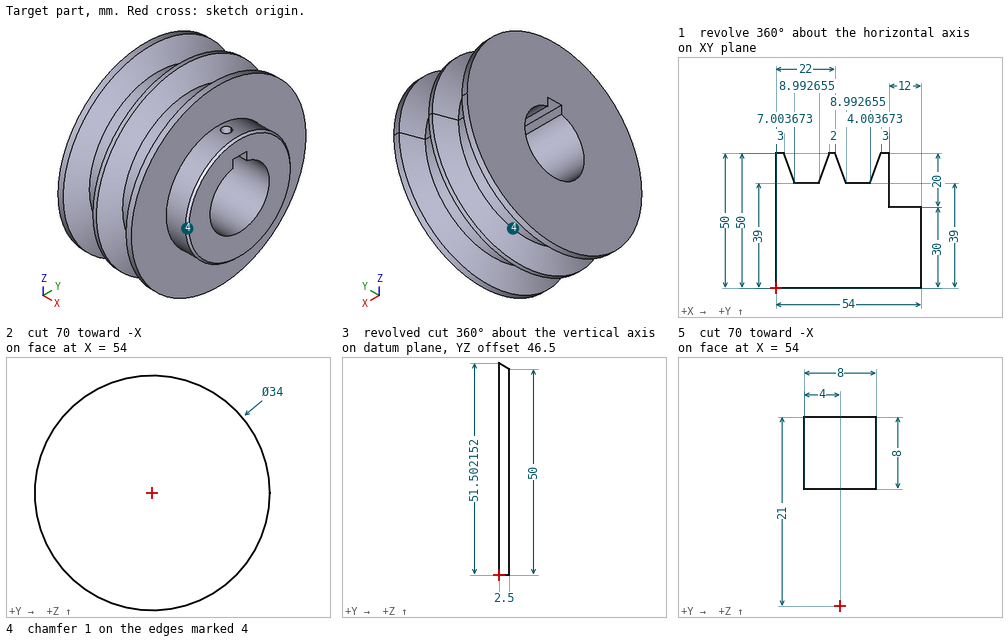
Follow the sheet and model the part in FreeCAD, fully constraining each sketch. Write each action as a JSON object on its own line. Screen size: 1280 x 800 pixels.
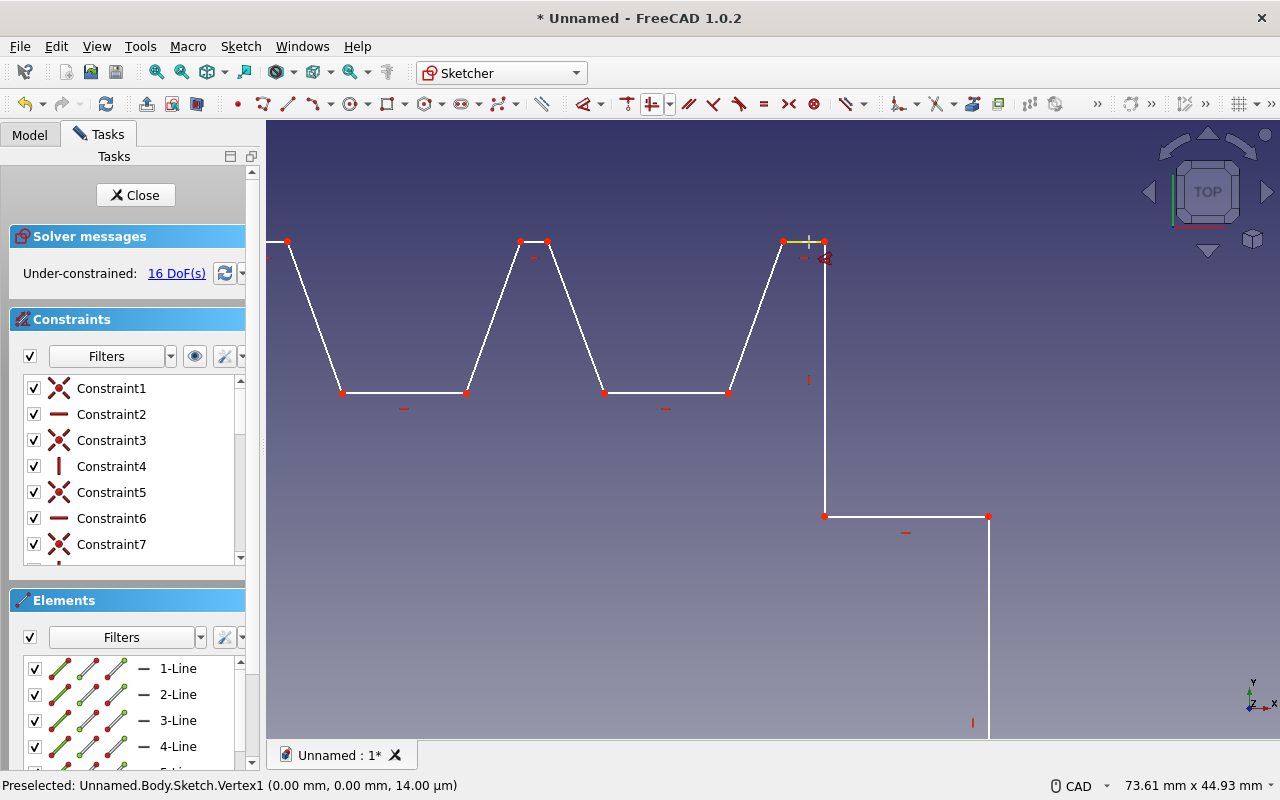
{"action": "left_click", "coordinate": [808, 242]}
{"action": "left_click", "coordinate": [804, 208]}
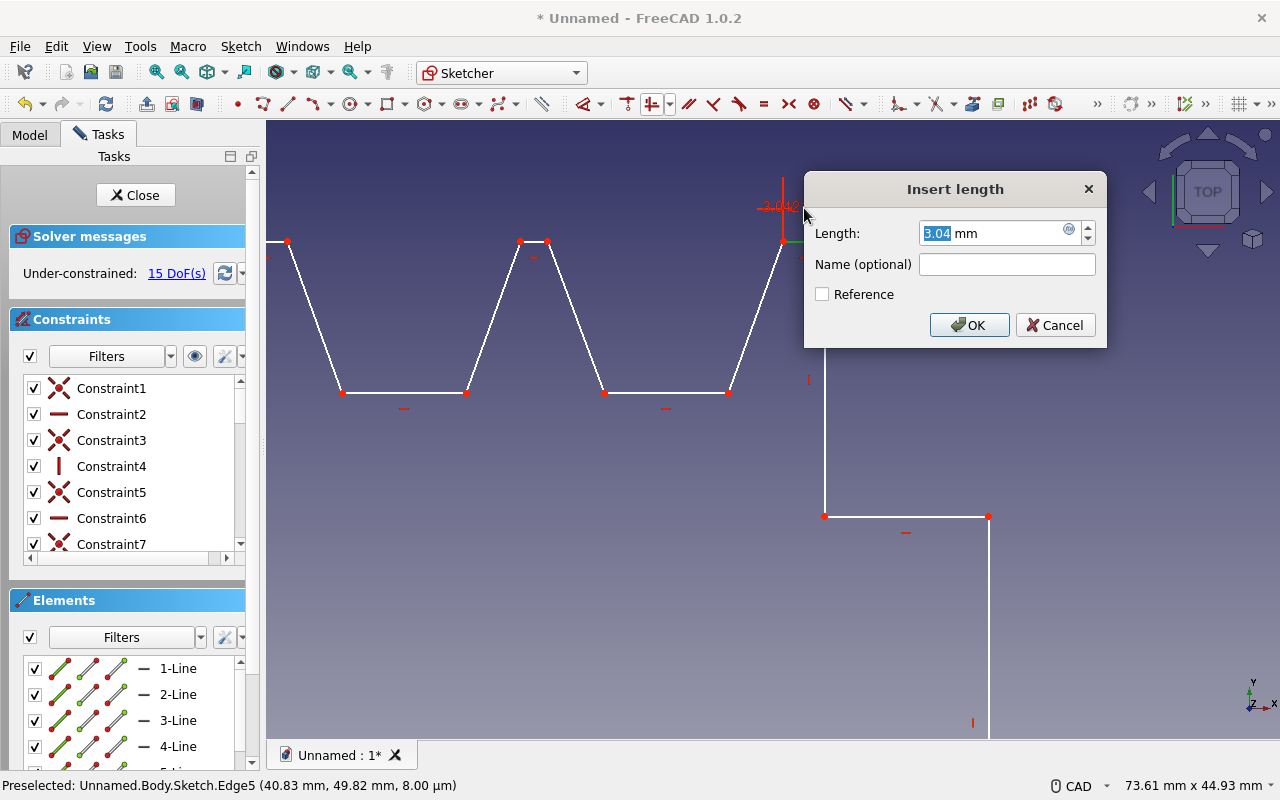
{"action": "type", "text": "3"}
{"action": "key", "text": "Return"}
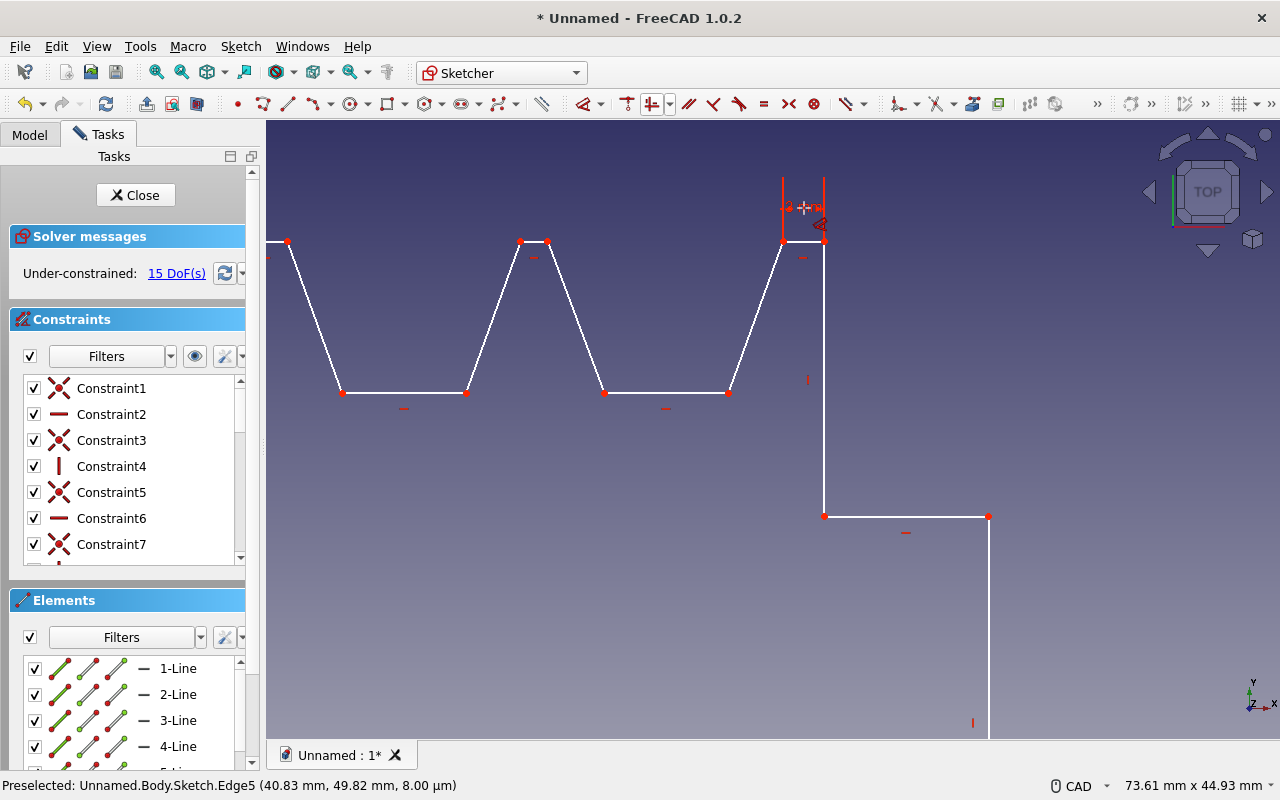
{"action": "scroll", "coordinate": [537, 242], "scroll_direction": "up", "scroll_amount": 2}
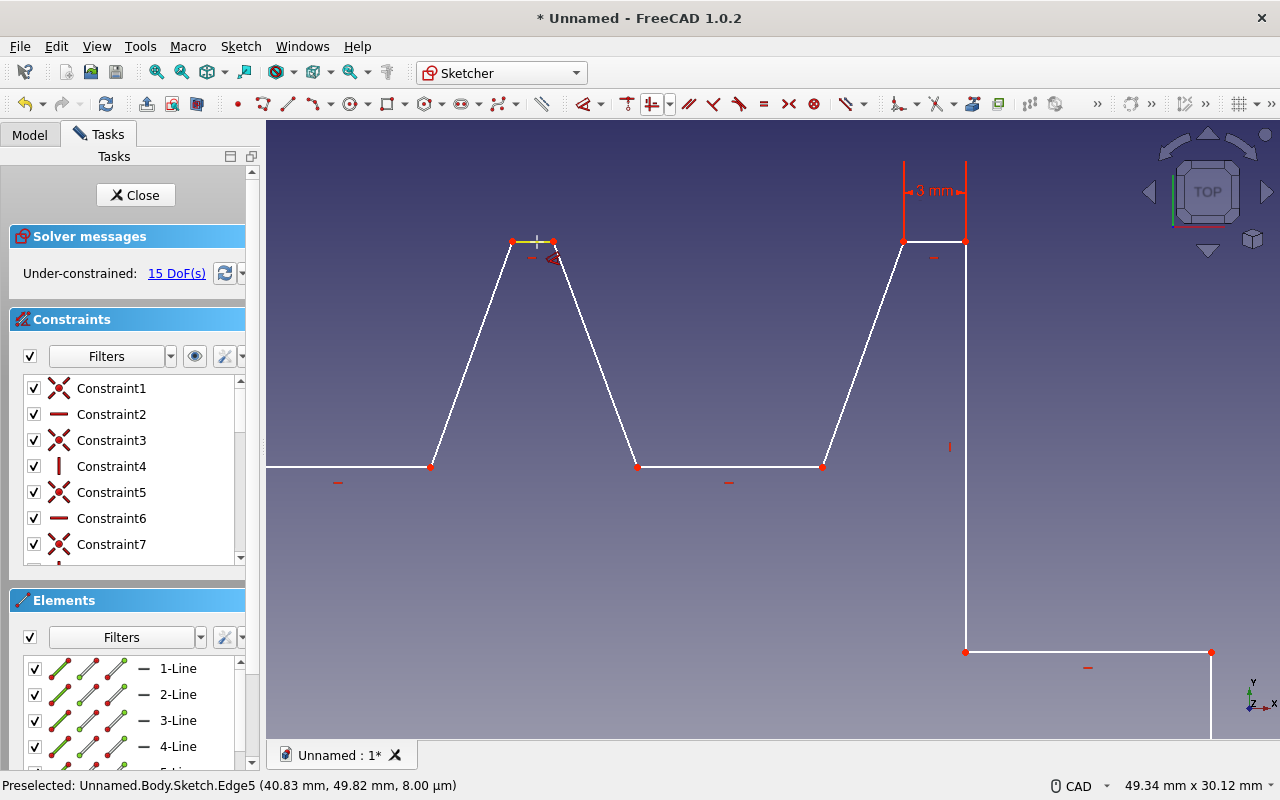
{"action": "left_click", "coordinate": [537, 242]}
{"action": "left_click", "coordinate": [533, 208]}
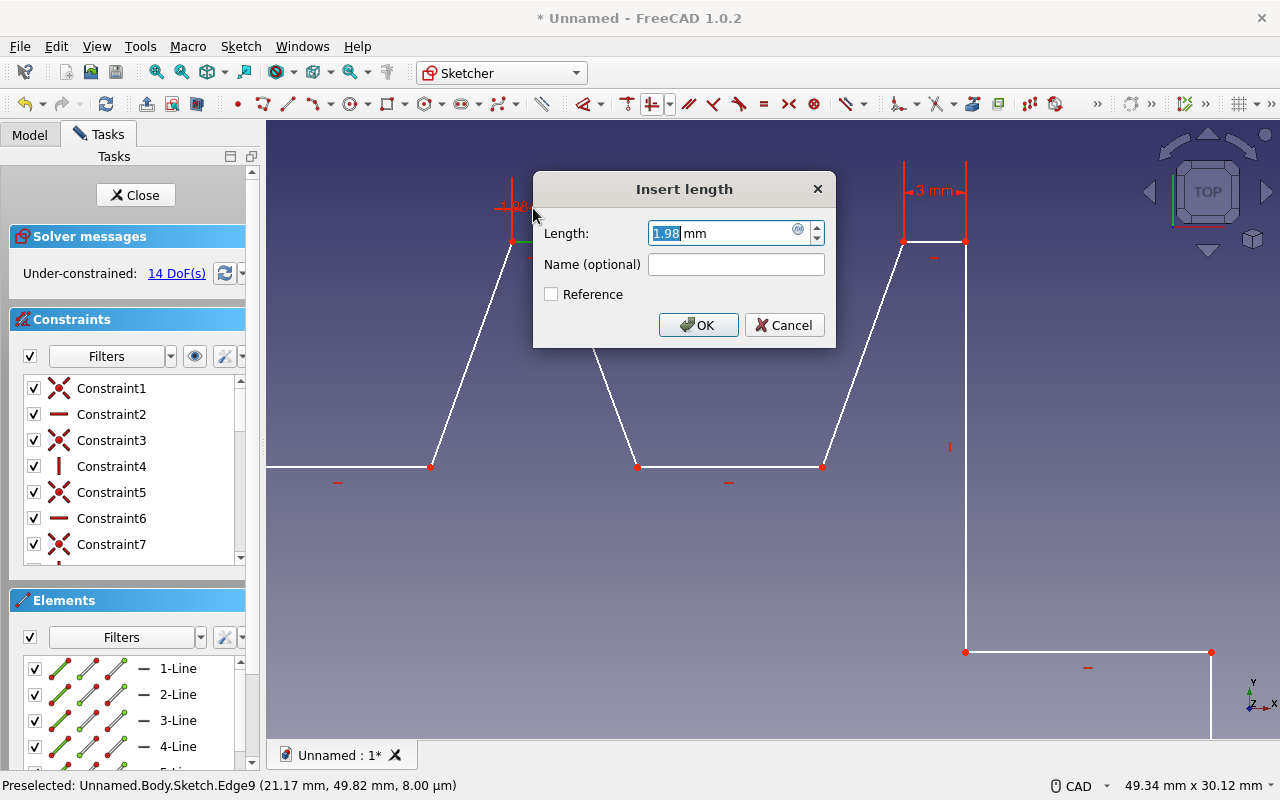
{"action": "type", "text": "2"}
{"action": "key", "text": "Return"}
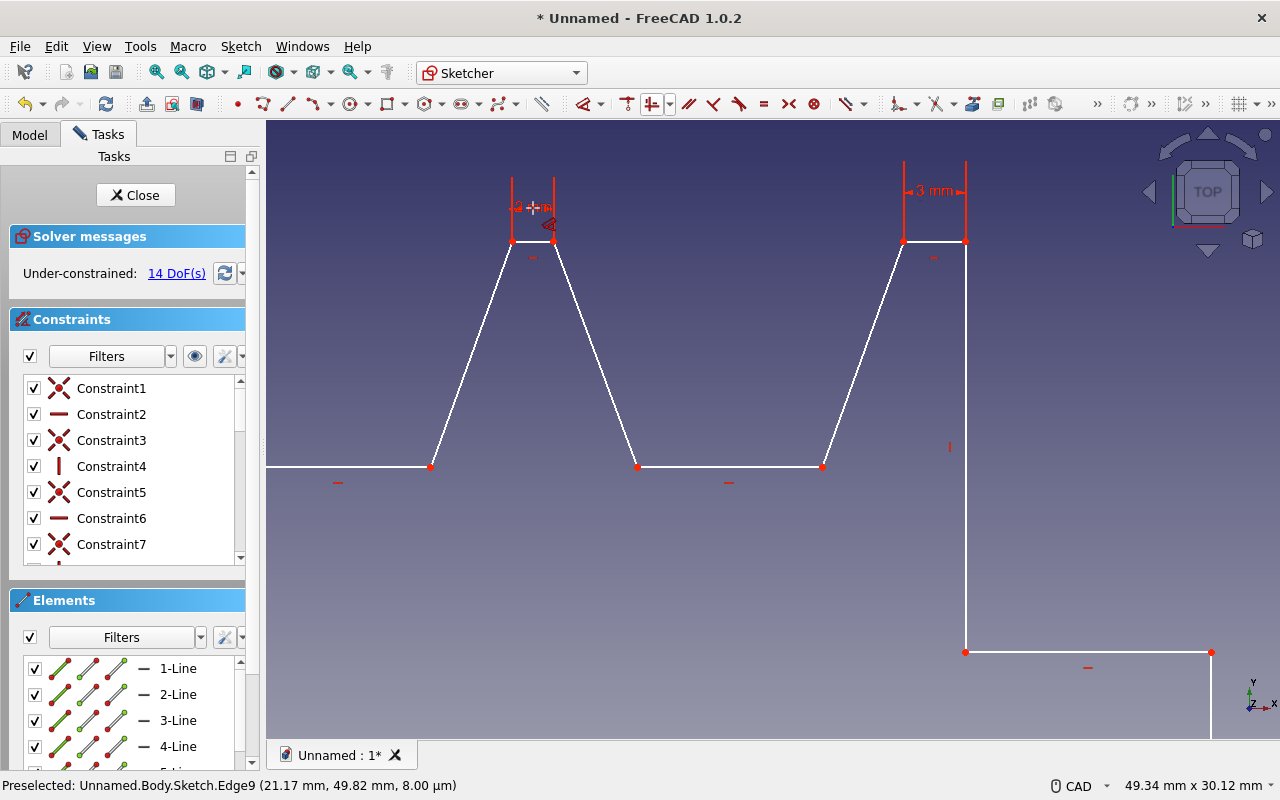
{"action": "scroll", "coordinate": [732, 242], "scroll_direction": "down", "scroll_amount": 5}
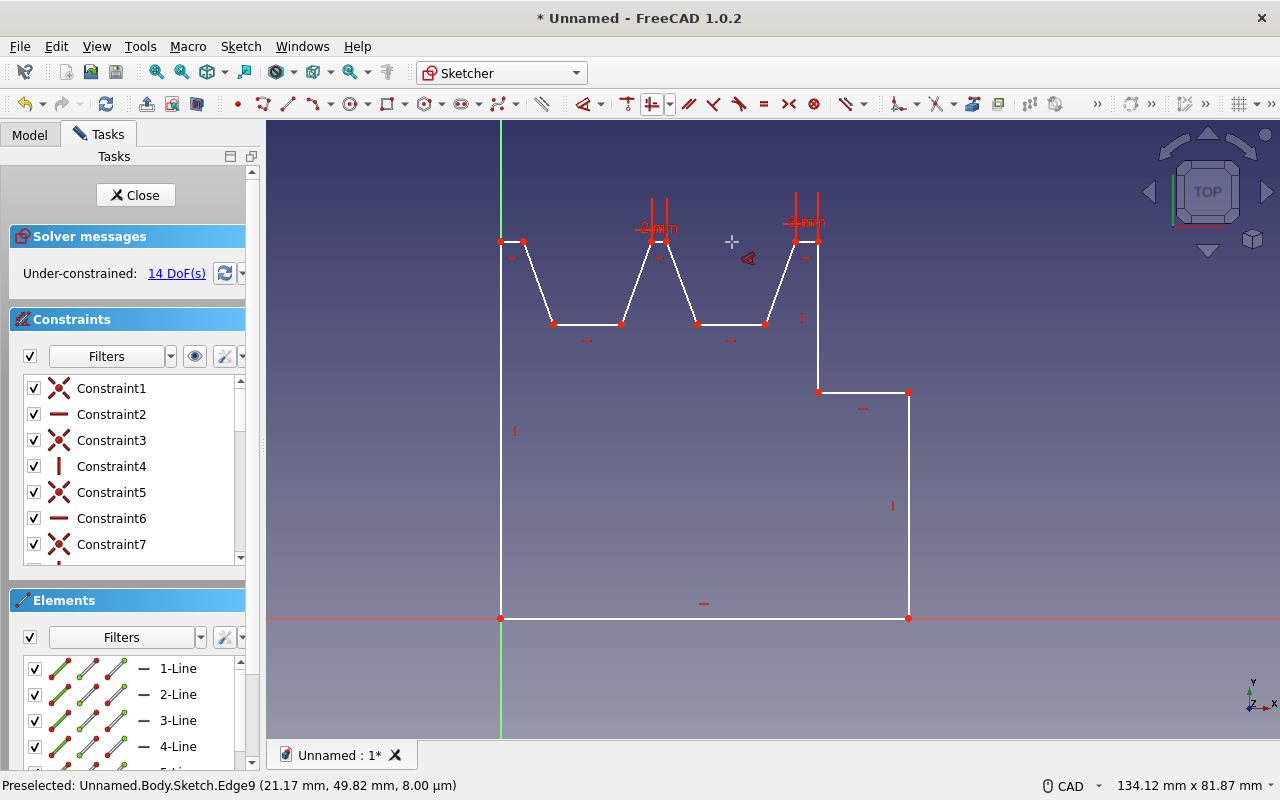
{"action": "scroll", "coordinate": [517, 242], "scroll_direction": "up", "scroll_amount": 4}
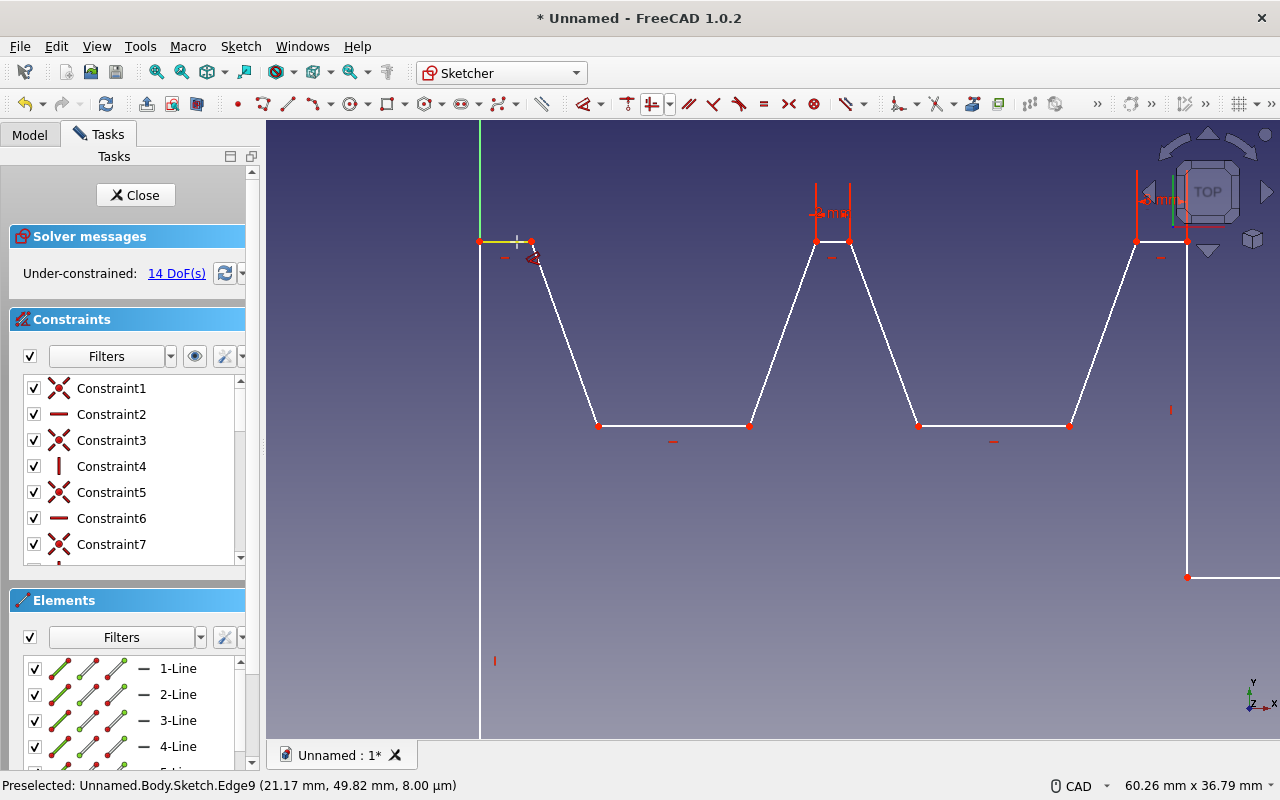
{"action": "left_click", "coordinate": [516, 242]}
{"action": "left_click", "coordinate": [506, 208]}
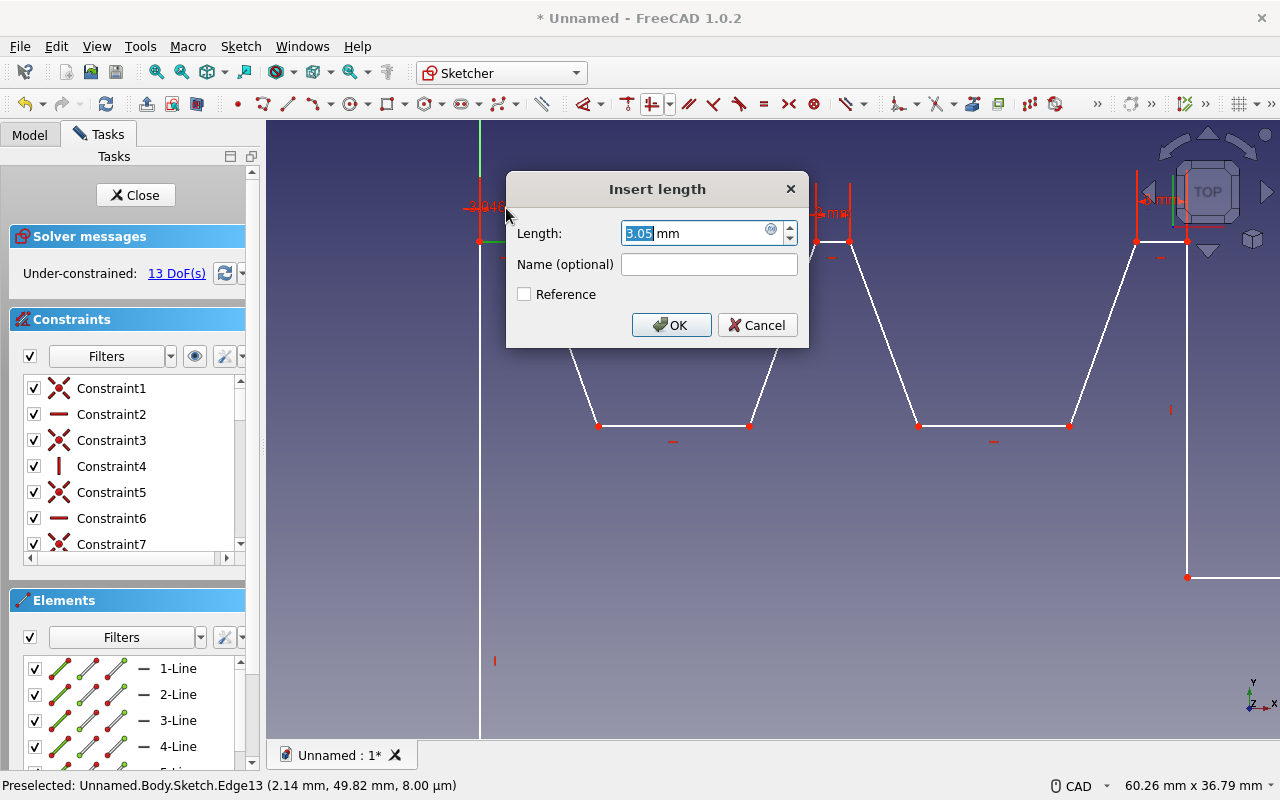
{"action": "type", "text": "3"}
{"action": "key", "text": "Return"}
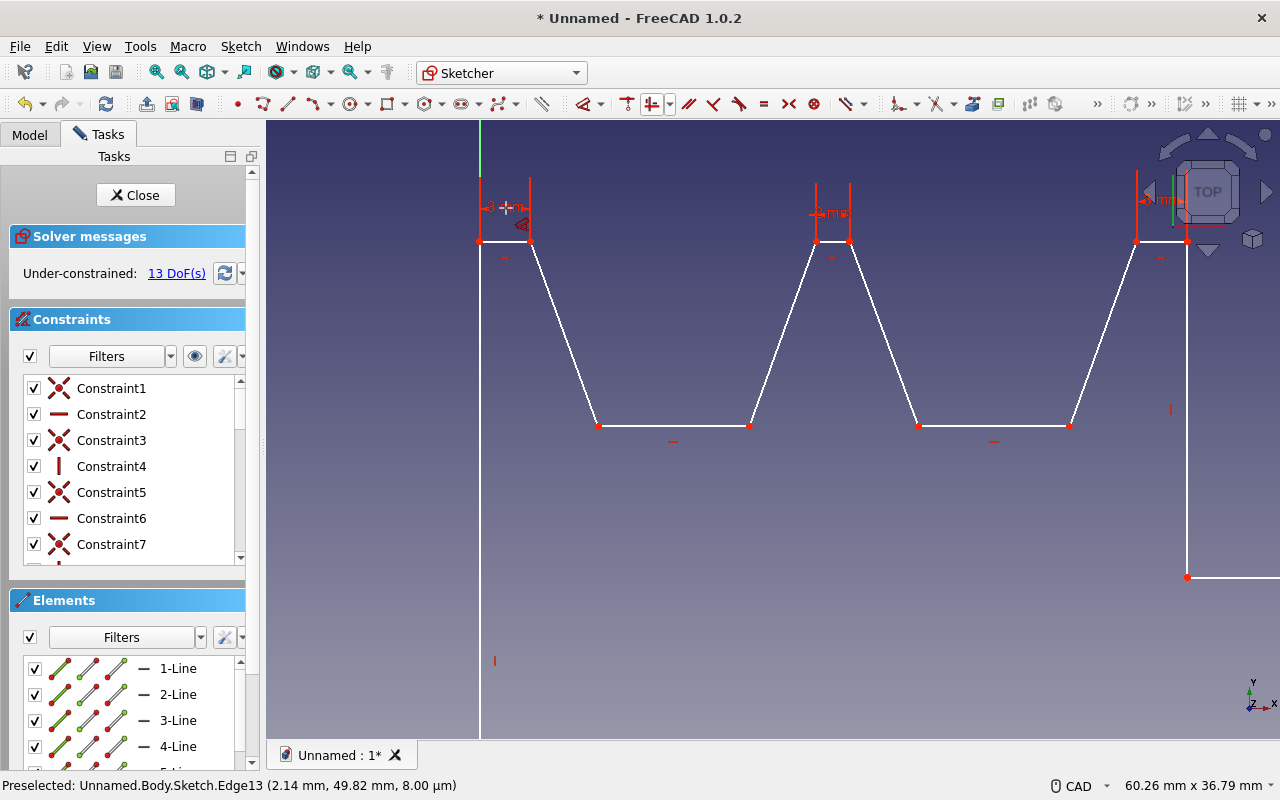
{"action": "scroll", "coordinate": [517, 242], "scroll_direction": "down", "scroll_amount": 4}